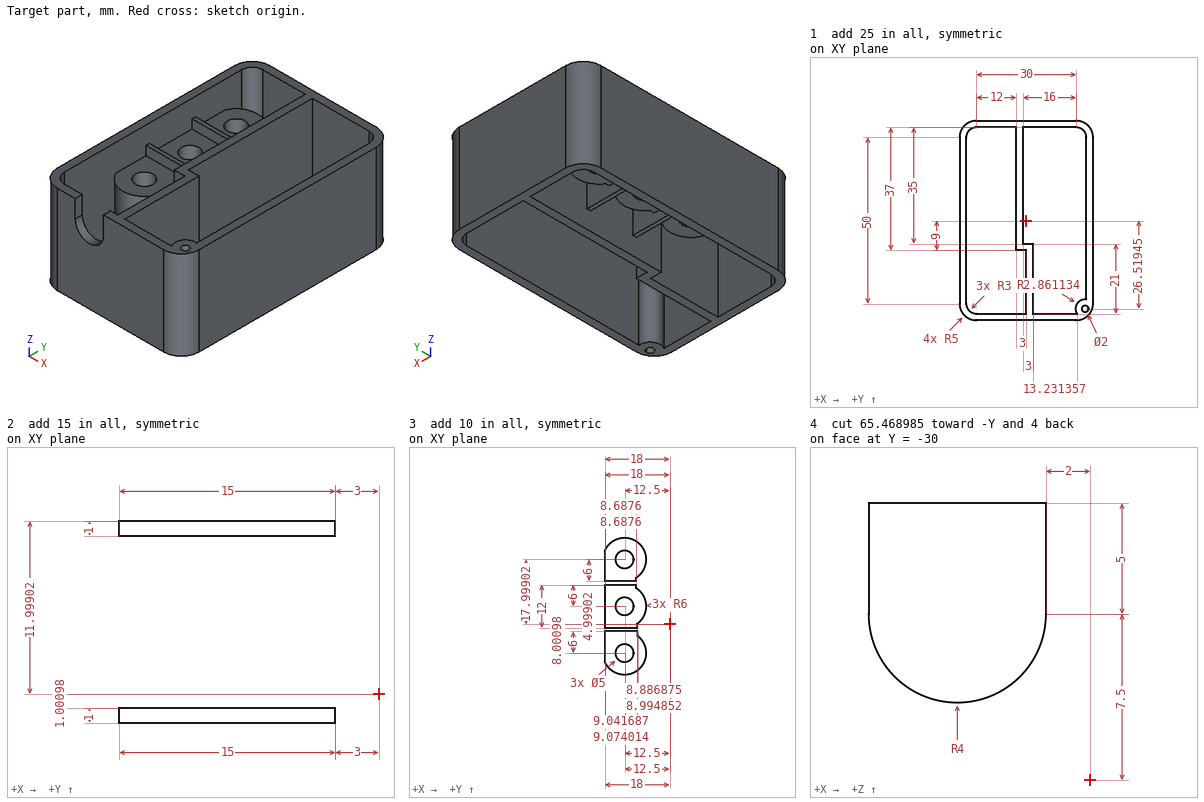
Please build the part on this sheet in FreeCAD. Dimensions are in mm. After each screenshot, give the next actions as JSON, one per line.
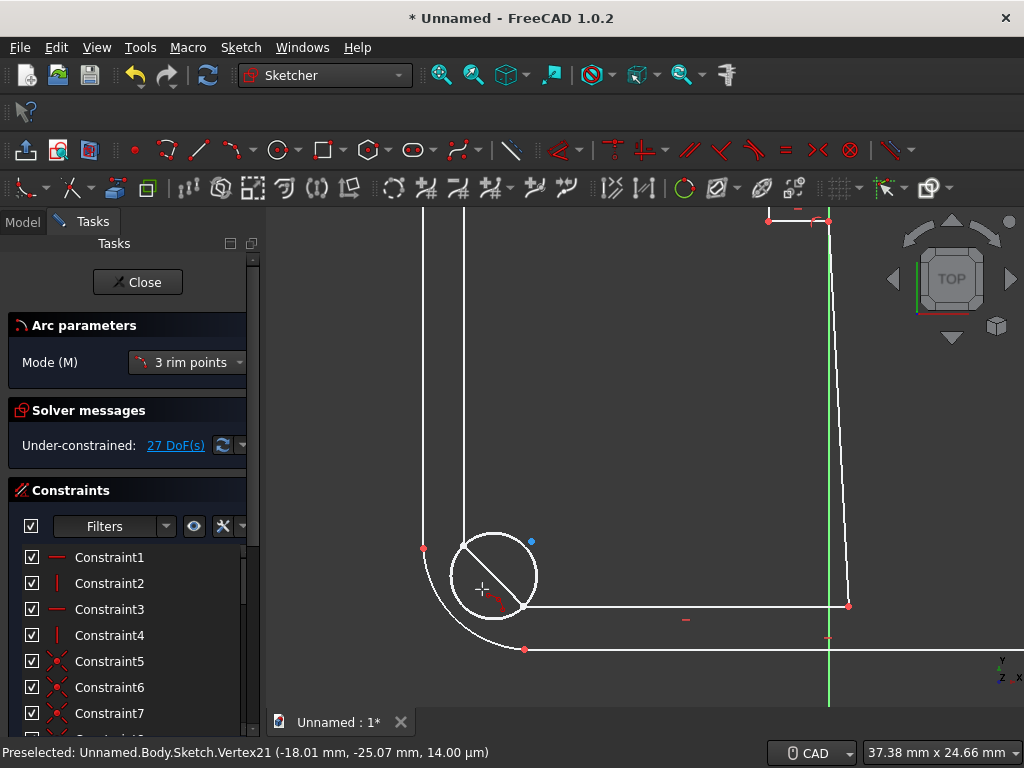
{"action": "left_click", "coordinate": [482, 587]}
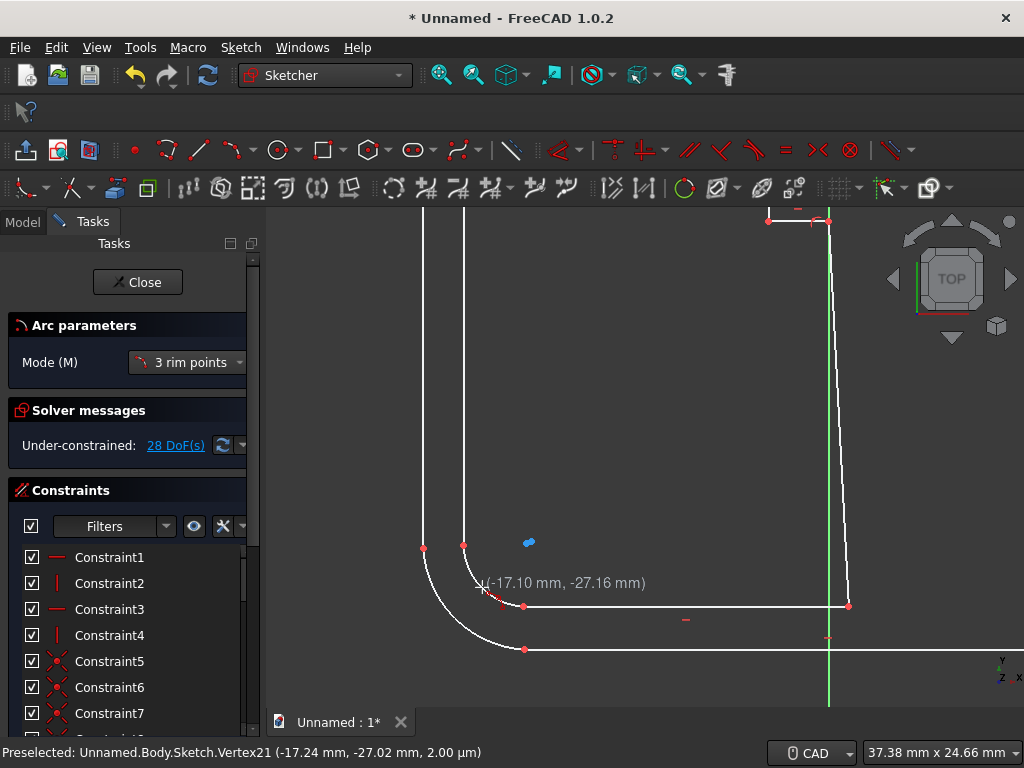
{"action": "left_click", "coordinate": [200, 150]}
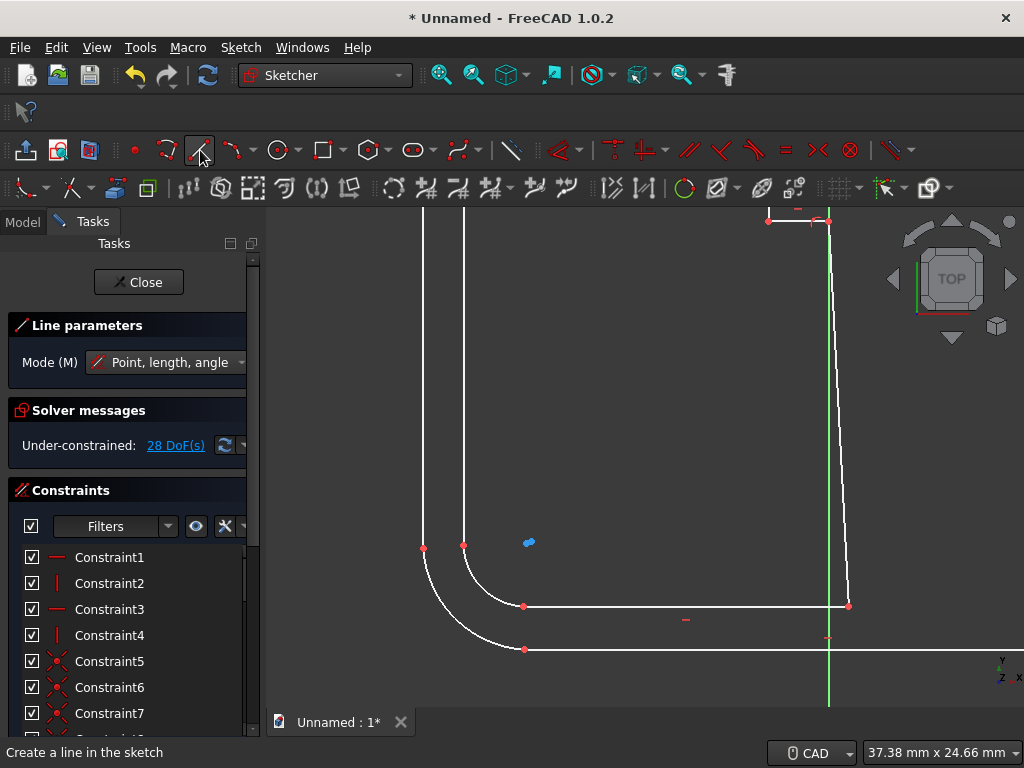
{"action": "scroll", "coordinate": [494, 594], "scroll_direction": "down", "scroll_amount": 7}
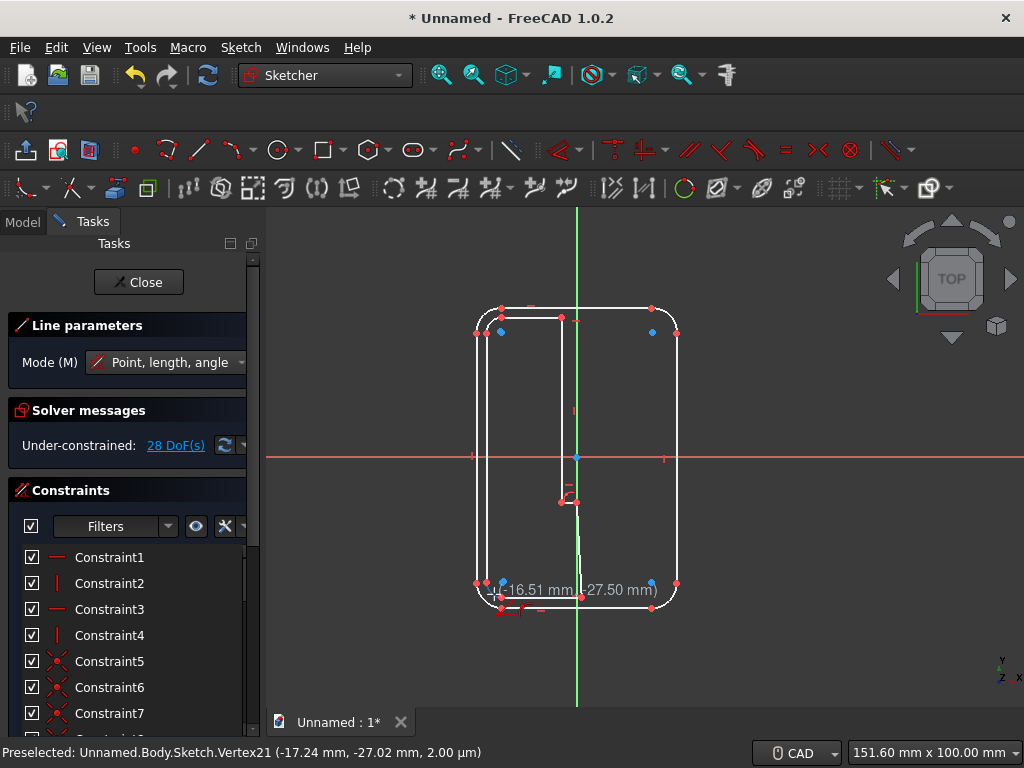
{"action": "scroll", "coordinate": [667, 332], "scroll_direction": "up", "scroll_amount": 3}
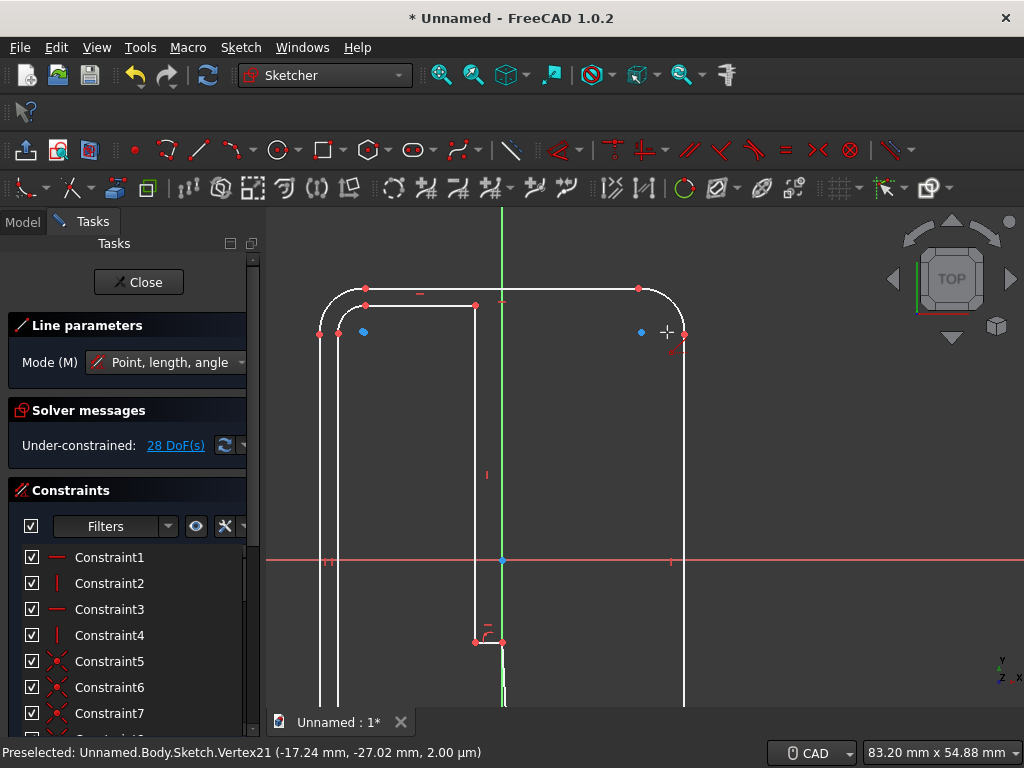
{"action": "left_click", "coordinate": [666, 332]}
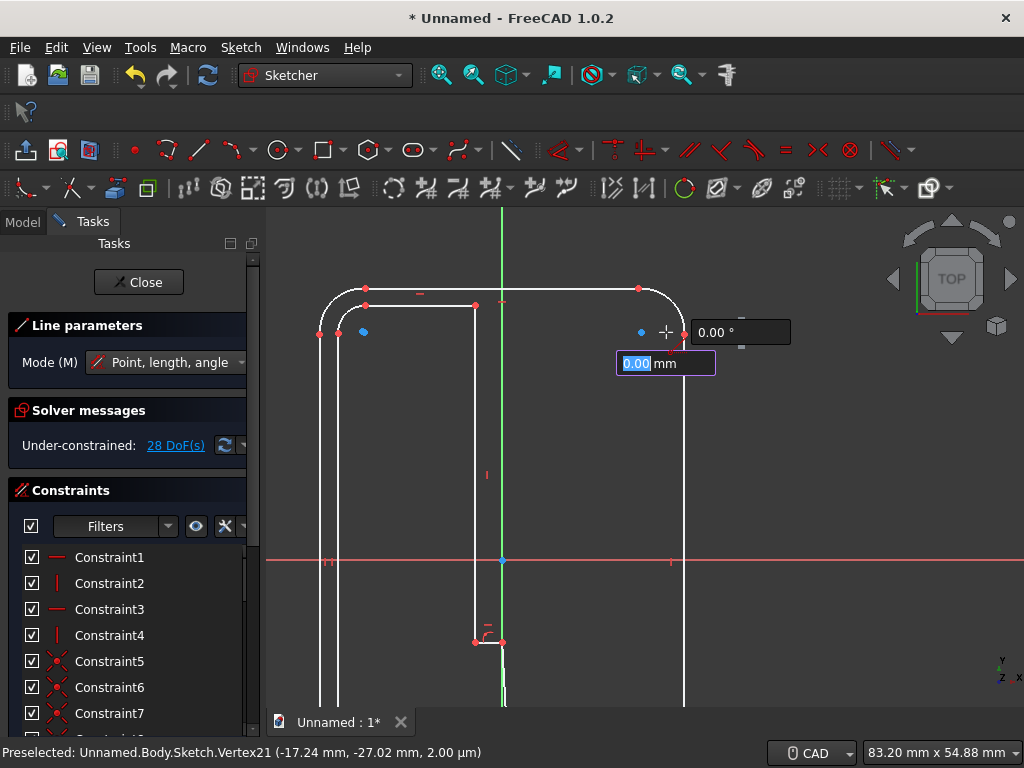
{"action": "scroll", "coordinate": [667, 332], "scroll_direction": "down", "scroll_amount": 3}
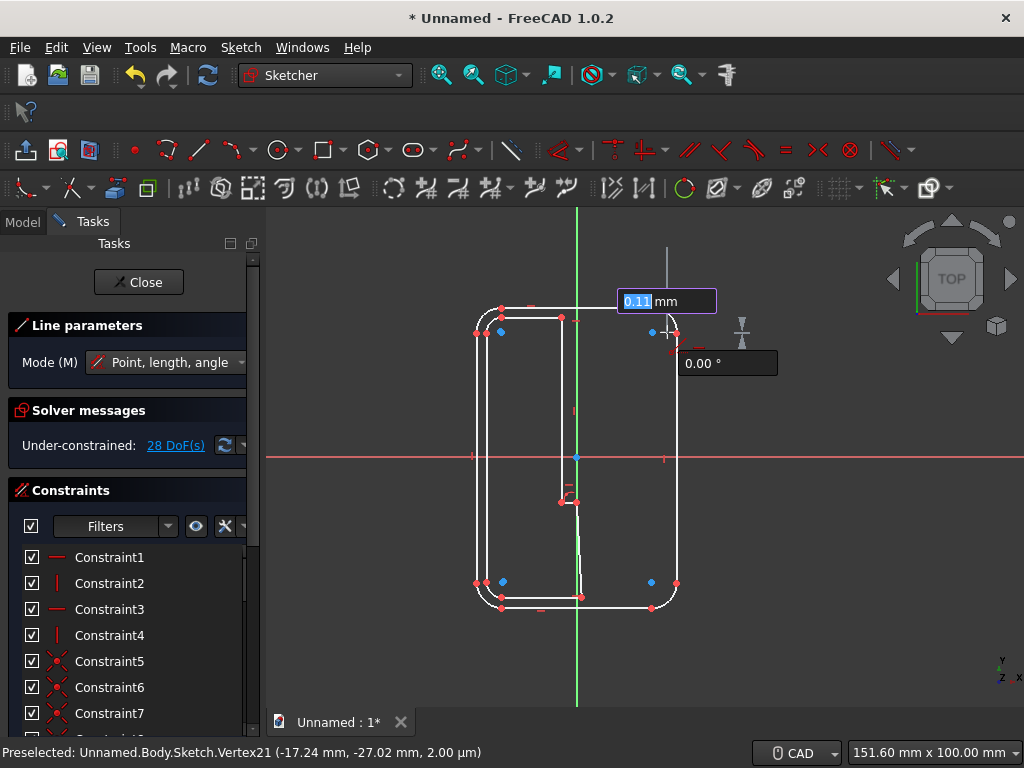
{"action": "scroll", "coordinate": [667, 576], "scroll_direction": "up", "scroll_amount": 3}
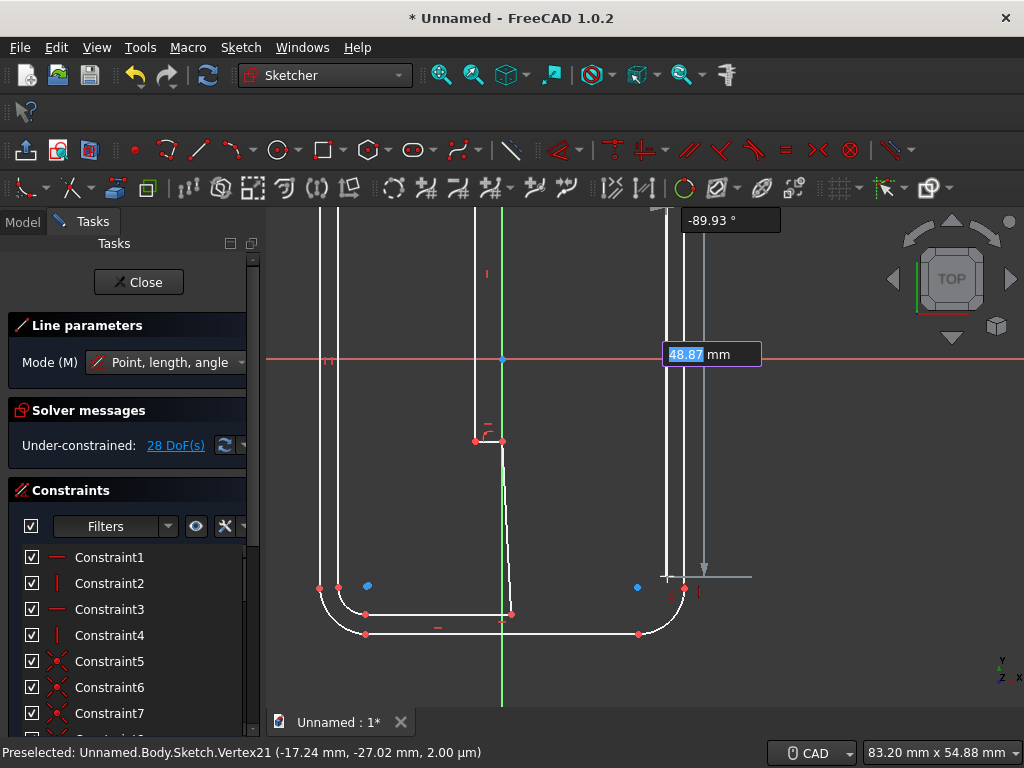
{"action": "left_click", "coordinate": [666, 575]}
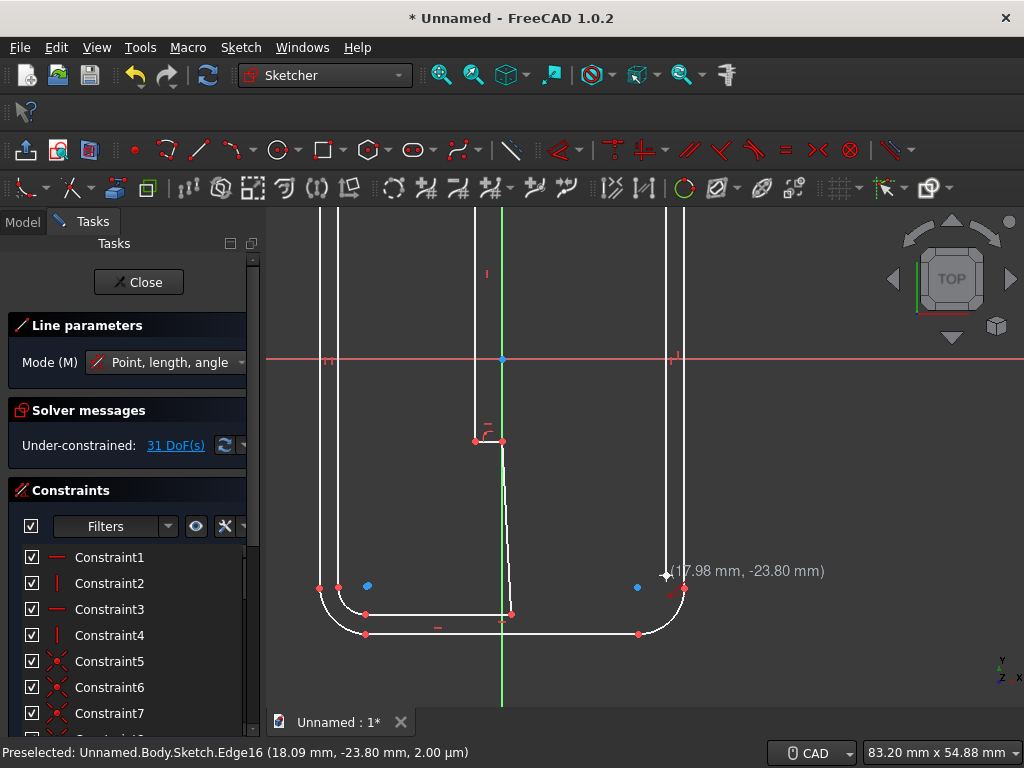
{"action": "left_click", "coordinate": [168, 150]}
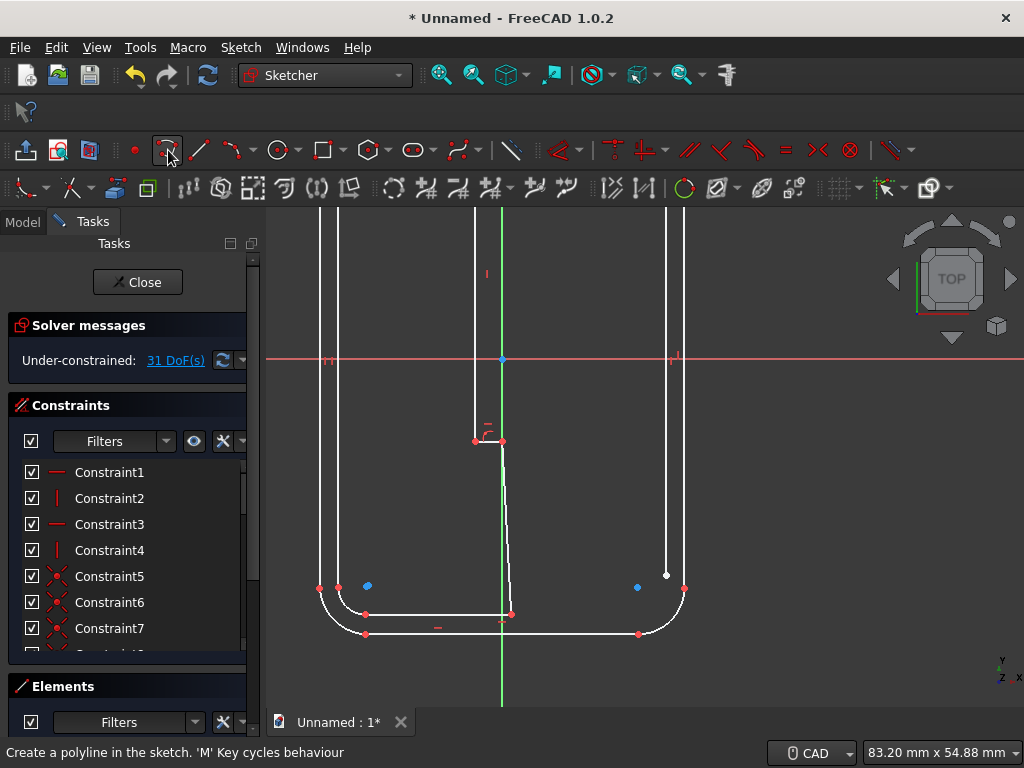
{"action": "left_click", "coordinate": [641, 614]}
{"action": "left_click", "coordinate": [520, 614]}
{"action": "left_click", "coordinate": [520, 423]}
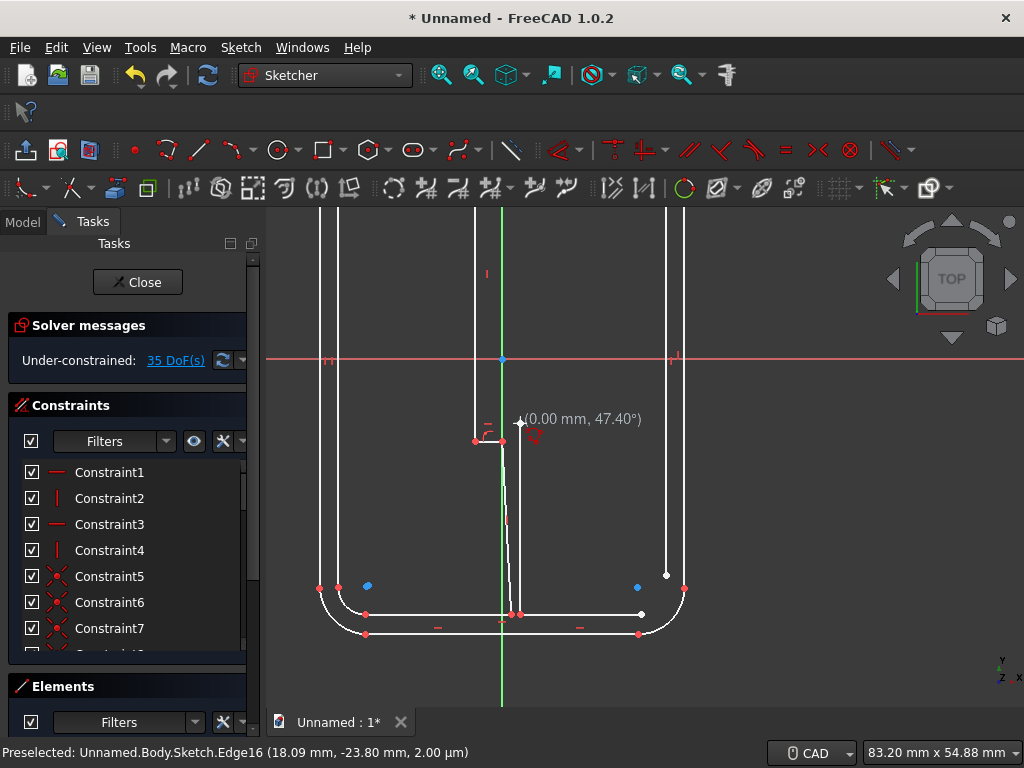
{"action": "scroll", "coordinate": [493, 423], "scroll_direction": "up", "scroll_amount": 3}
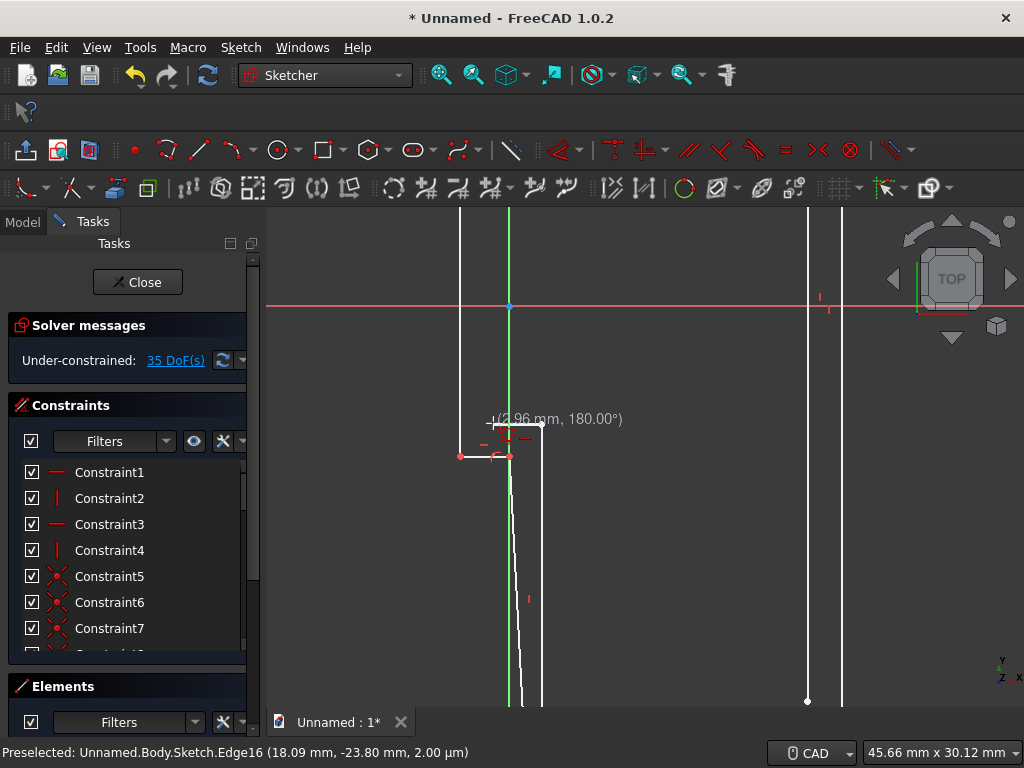
{"action": "left_click", "coordinate": [493, 423]}